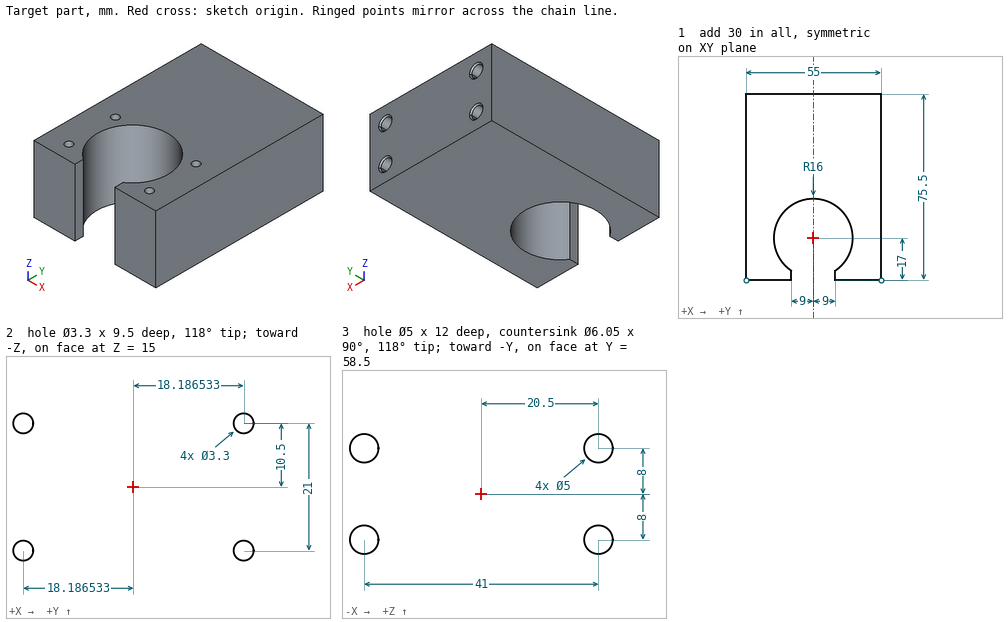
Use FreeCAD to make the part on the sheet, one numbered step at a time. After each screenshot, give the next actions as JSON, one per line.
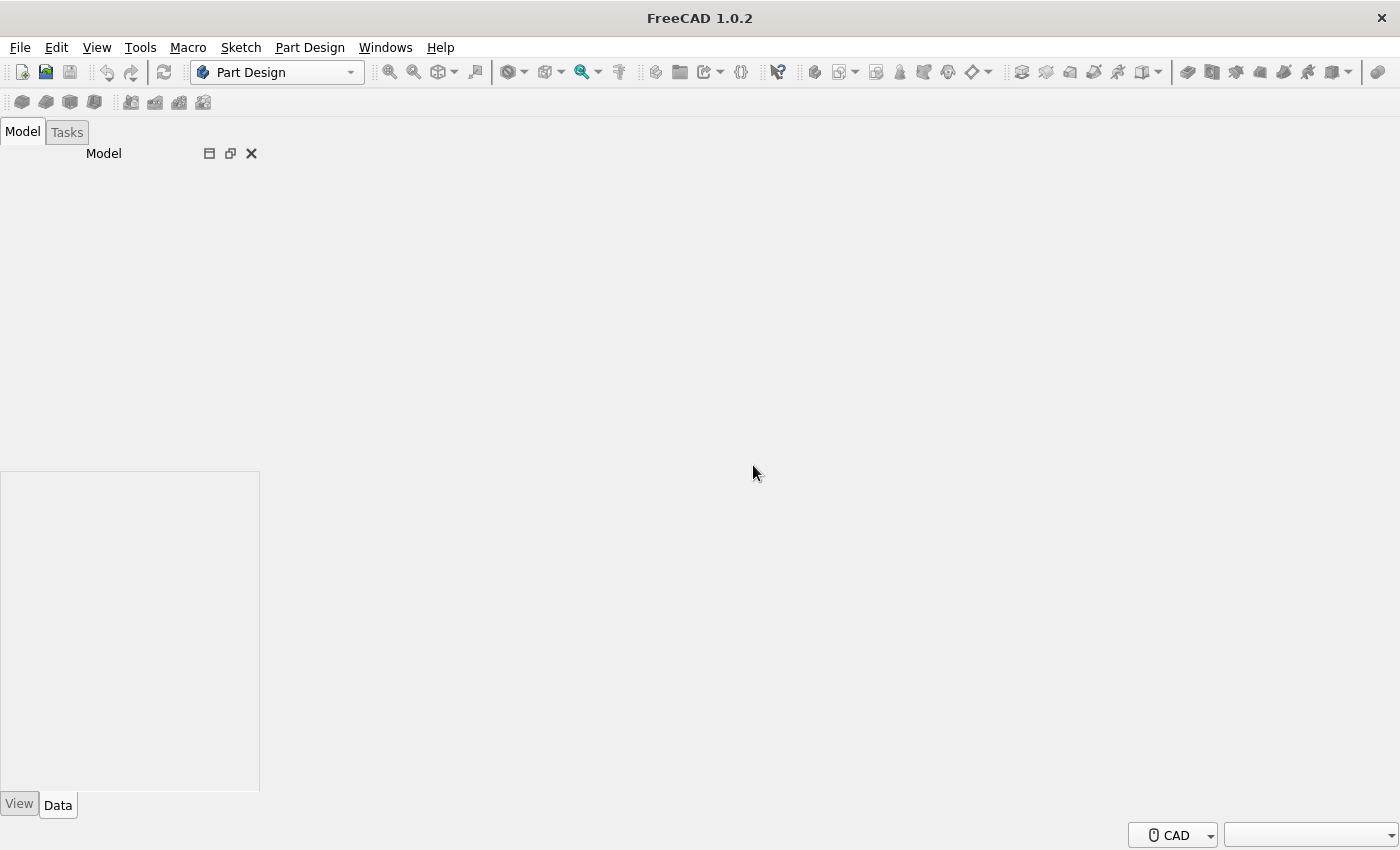
{"action": "left_click", "coordinate": [22, 72]}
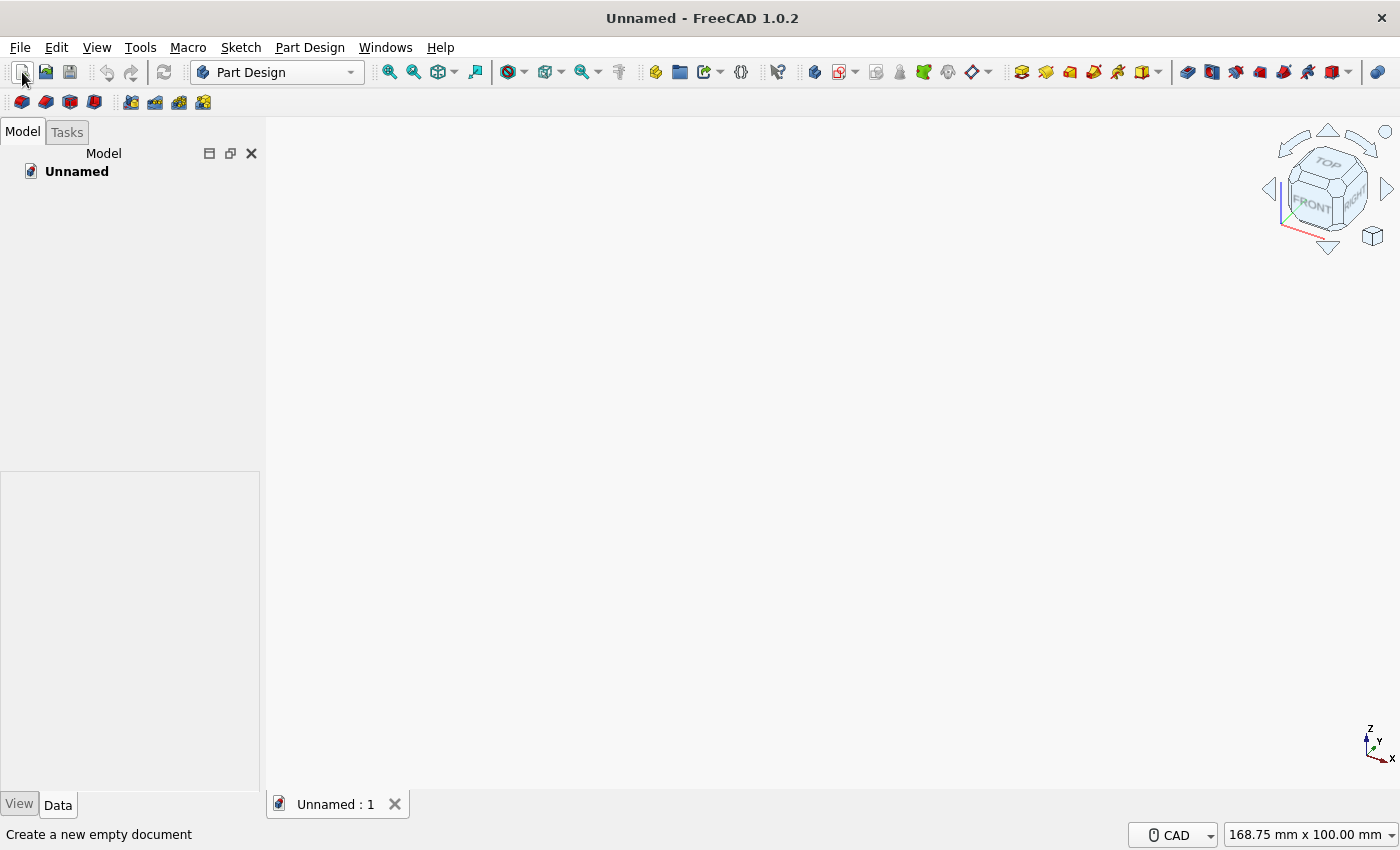
{"action": "left_click", "coordinate": [840, 72]}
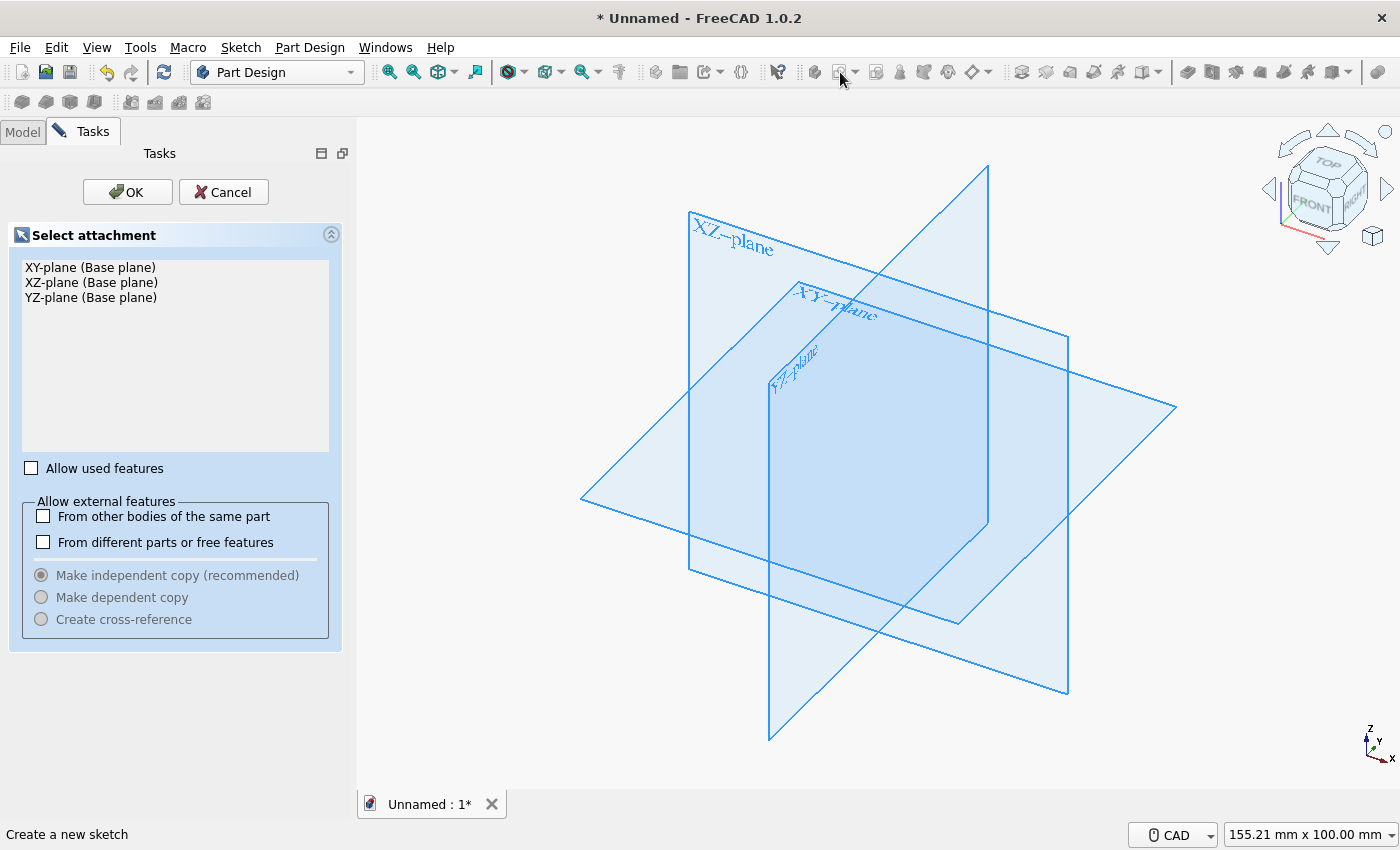
{"action": "left_click", "coordinate": [82, 268]}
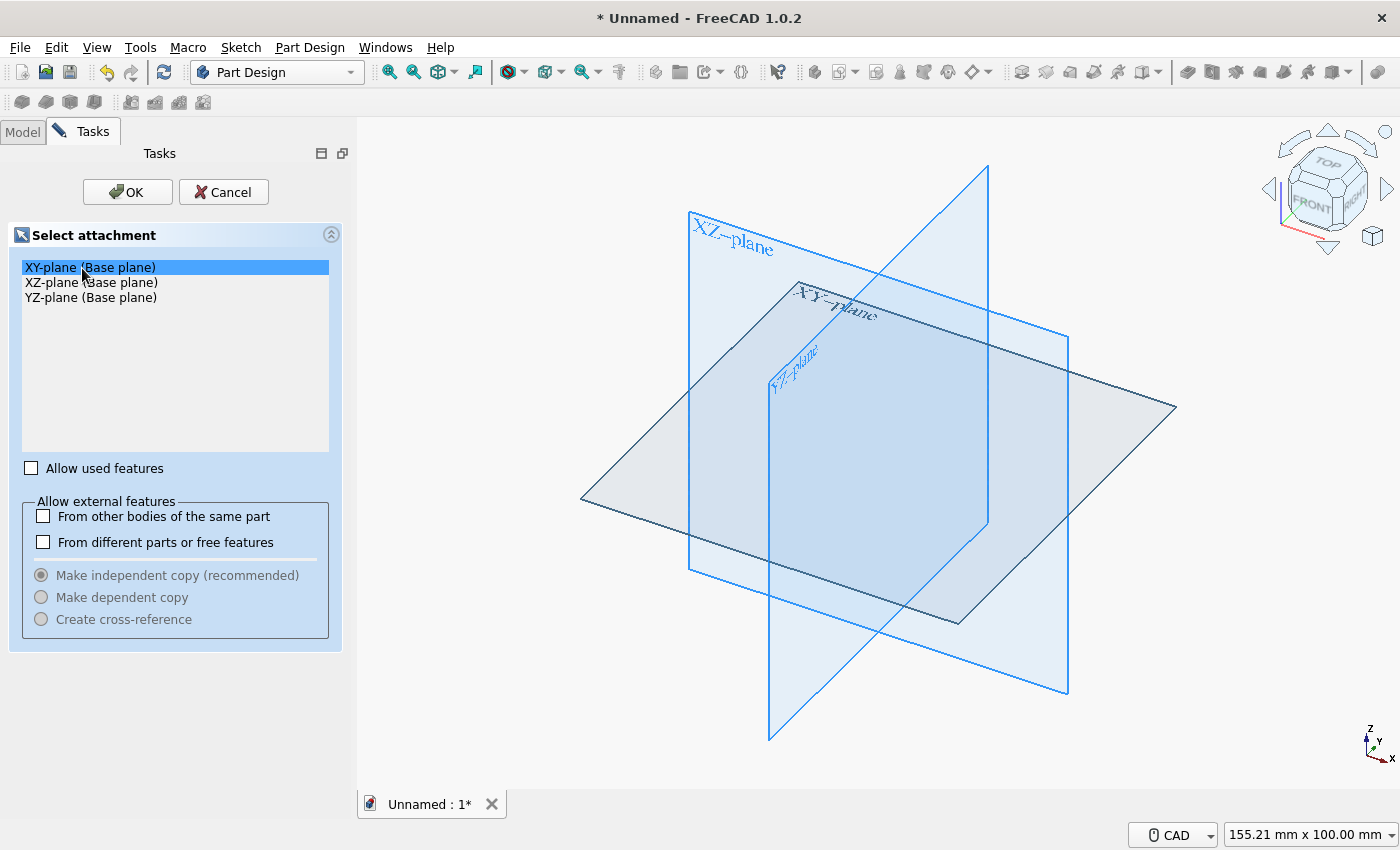
{"action": "left_click", "coordinate": [128, 192]}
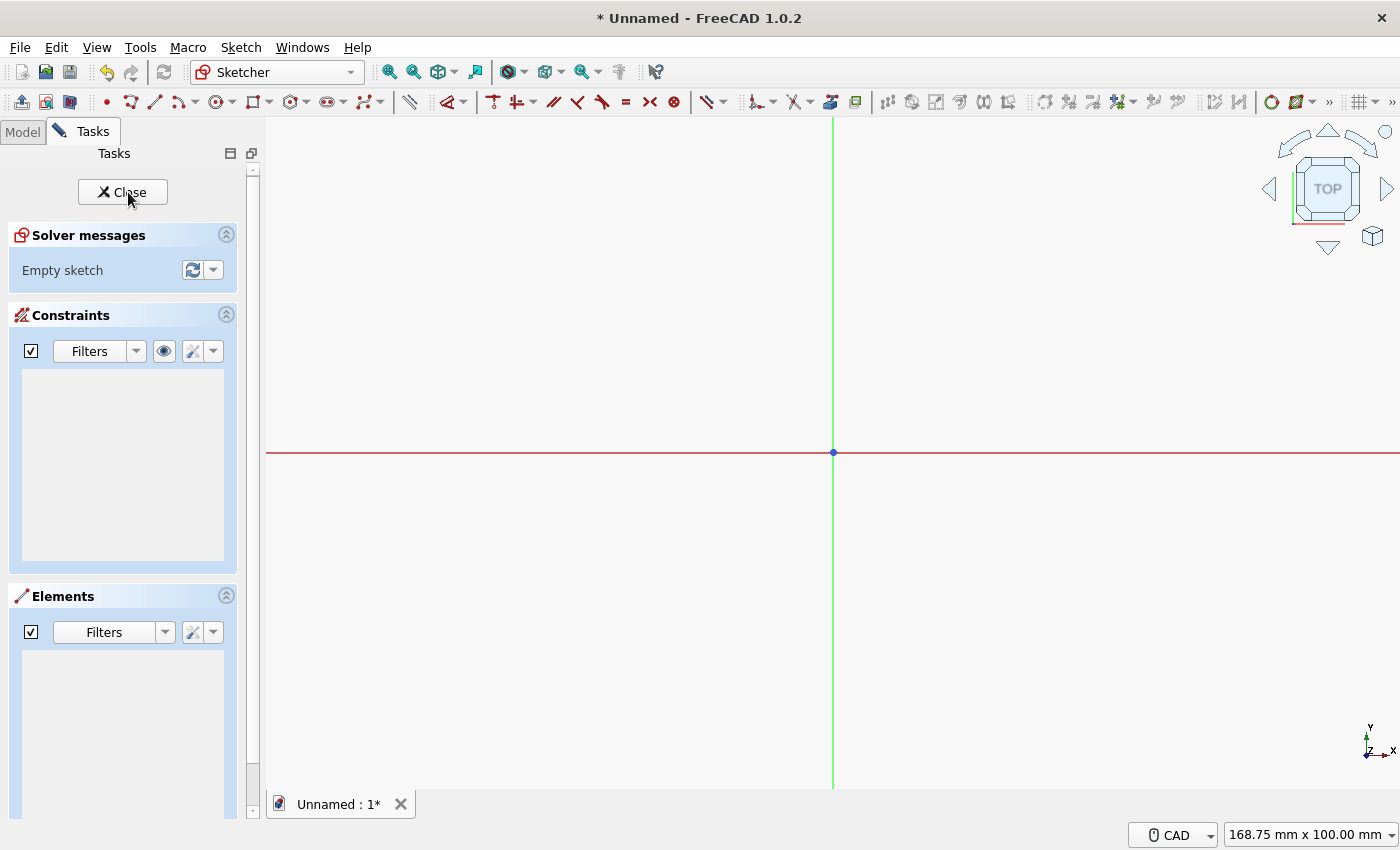
{"action": "scroll", "coordinate": [455, 761], "scroll_direction": "down", "scroll_amount": 1}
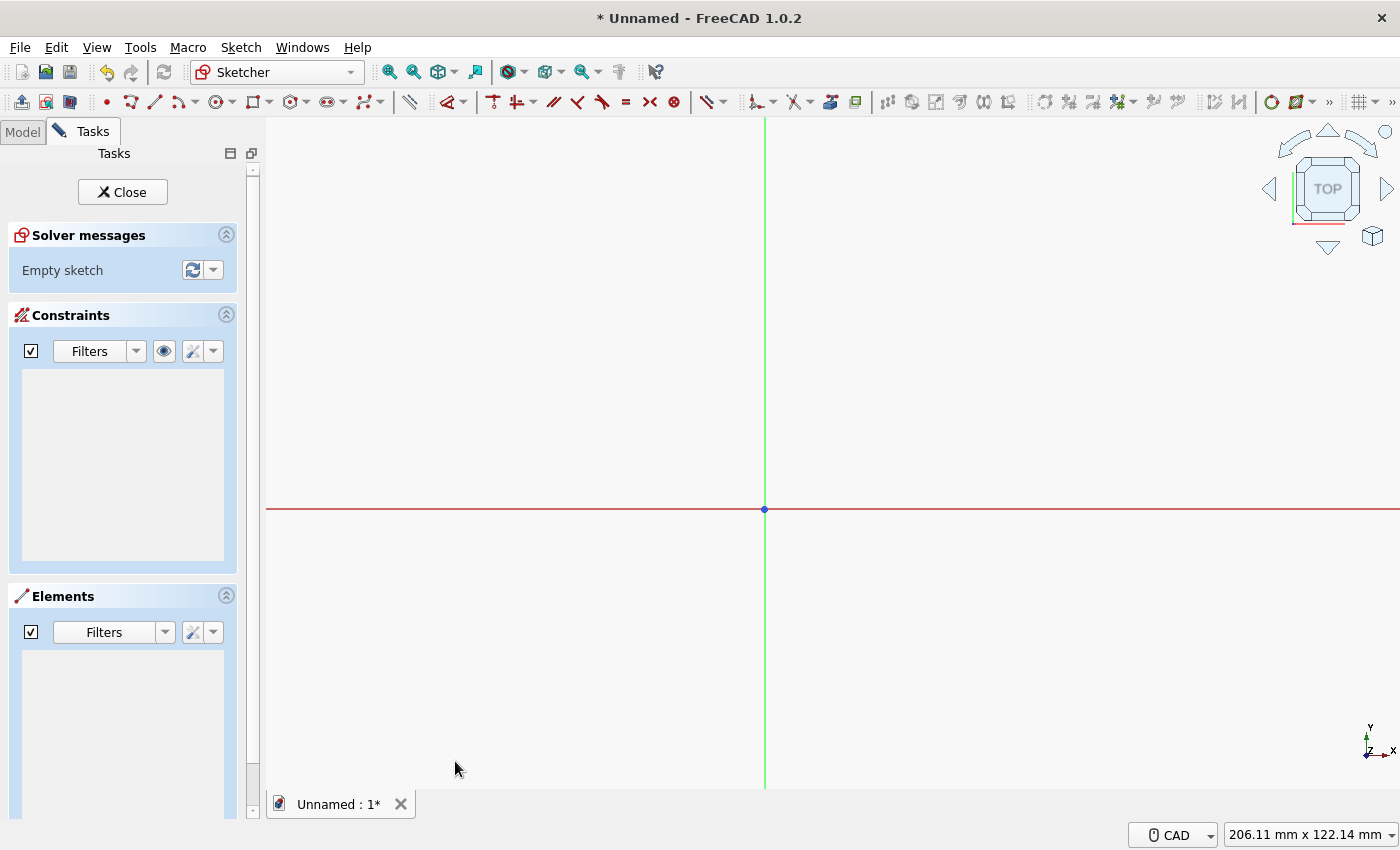
{"action": "left_click", "coordinate": [132, 102]}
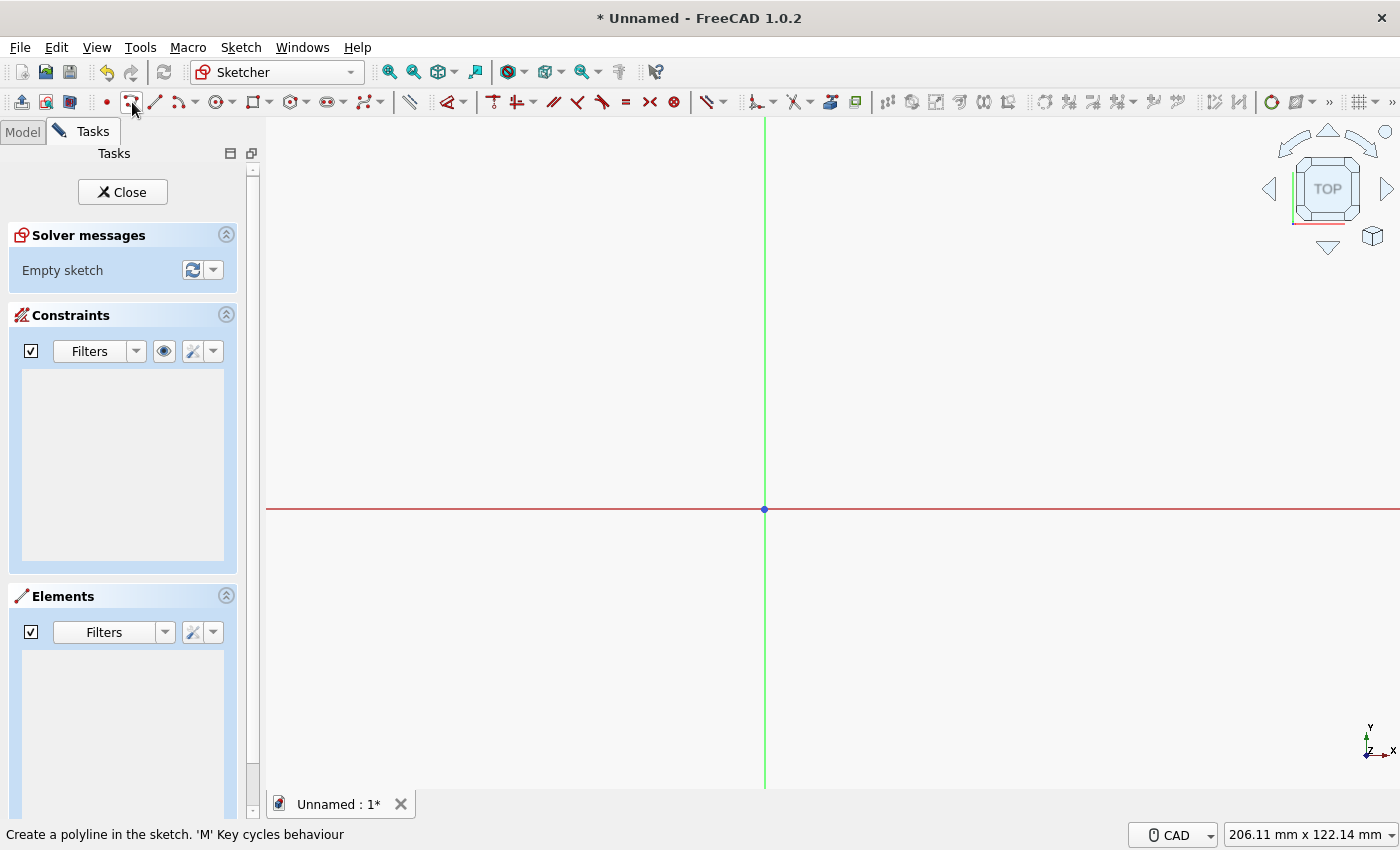
{"action": "left_click", "coordinate": [814, 582]}
{"action": "left_click", "coordinate": [814, 603]}
{"action": "left_click", "coordinate": [916, 603]}
{"action": "left_click", "coordinate": [916, 187]}
{"action": "left_click", "coordinate": [613, 187]}
{"action": "left_click", "coordinate": [613, 603]}
{"action": "left_click", "coordinate": [715, 603]}
{"action": "left_click", "coordinate": [715, 582]}
{"action": "right_click", "coordinate": [715, 582]}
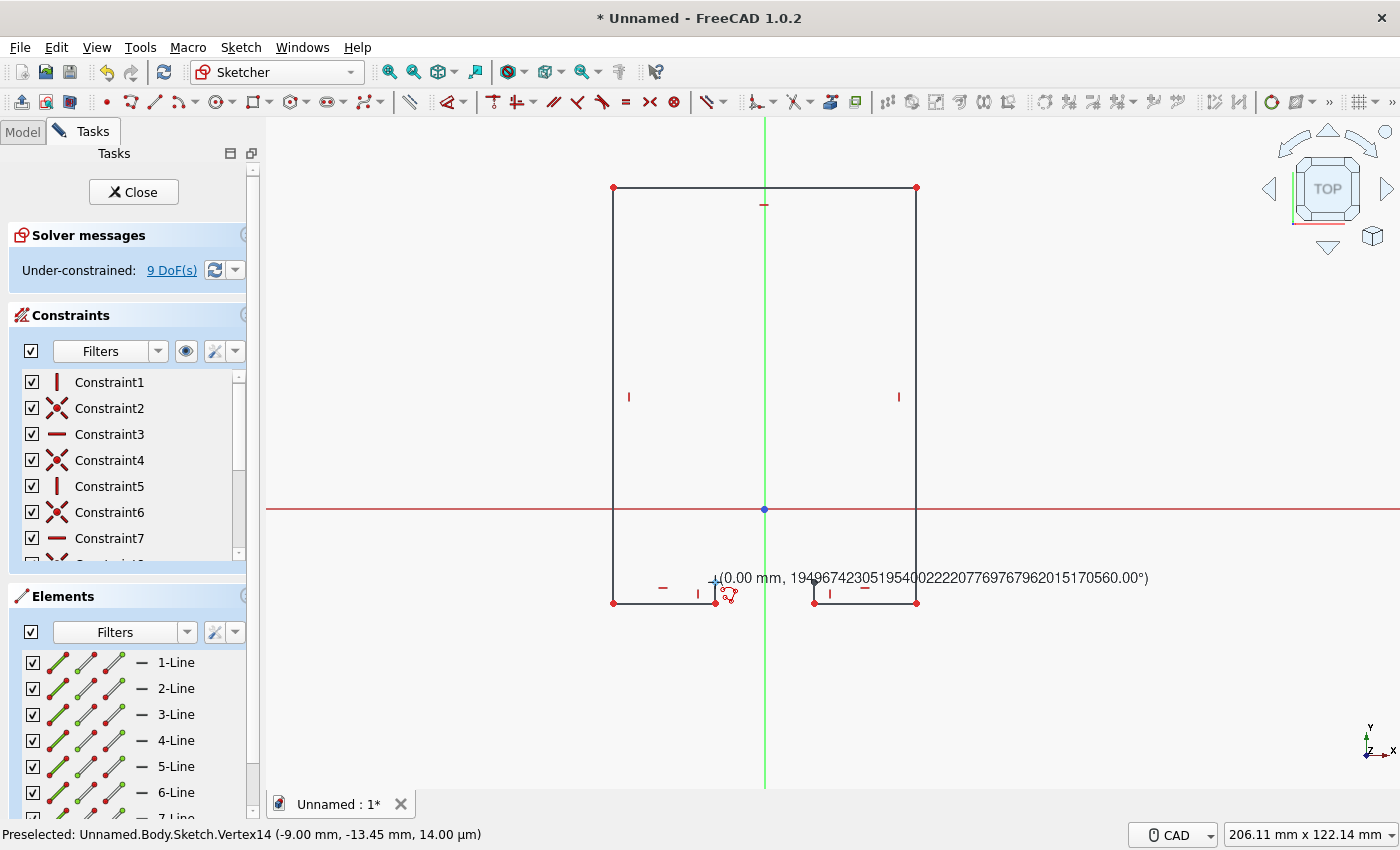
{"action": "left_click", "coordinate": [198, 102]}